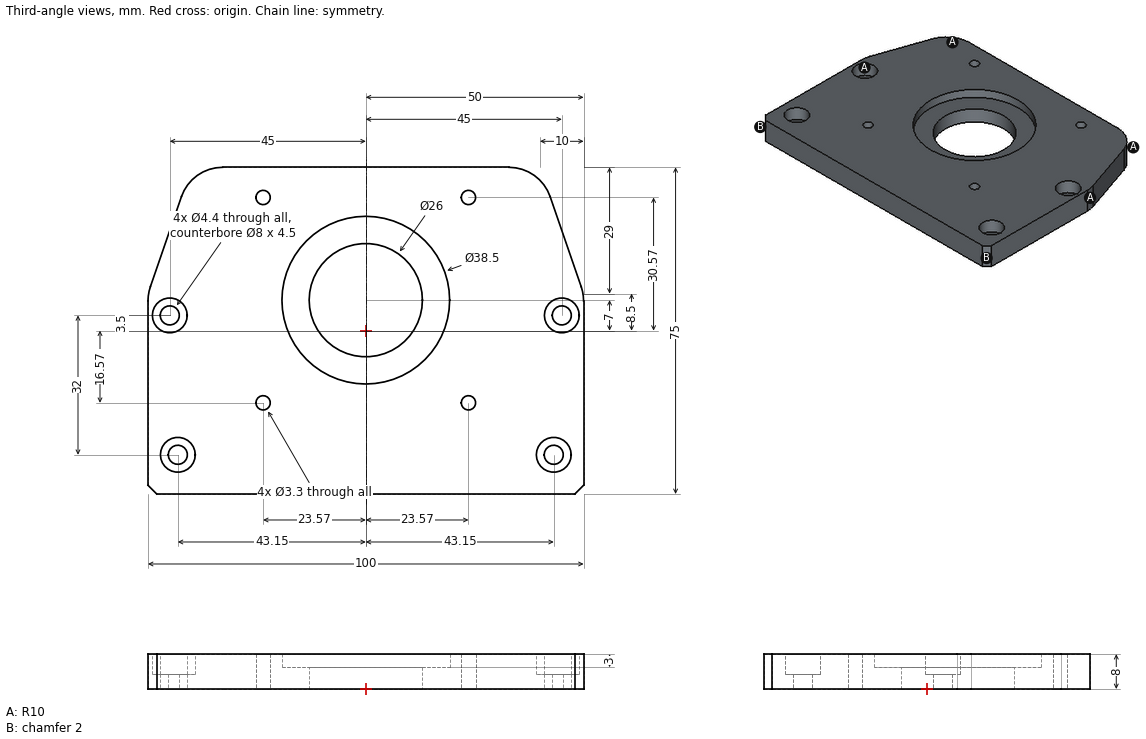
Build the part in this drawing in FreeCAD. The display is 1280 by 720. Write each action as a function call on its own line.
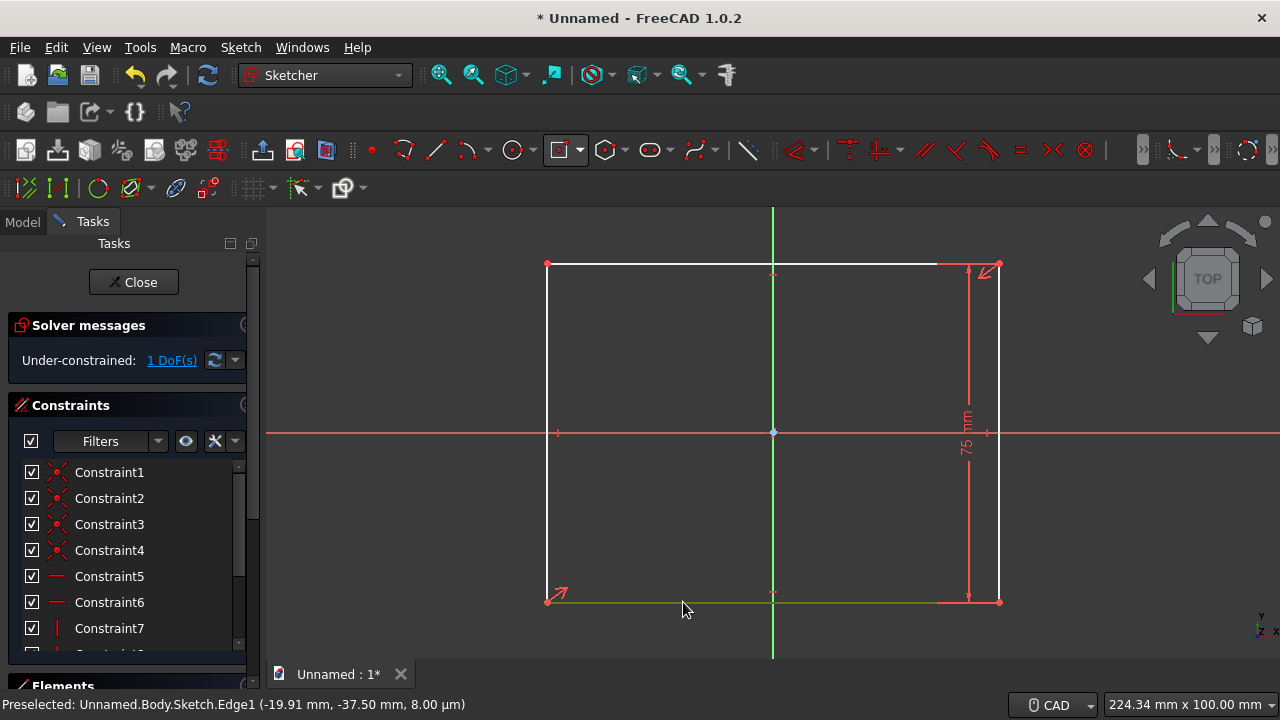
key(l)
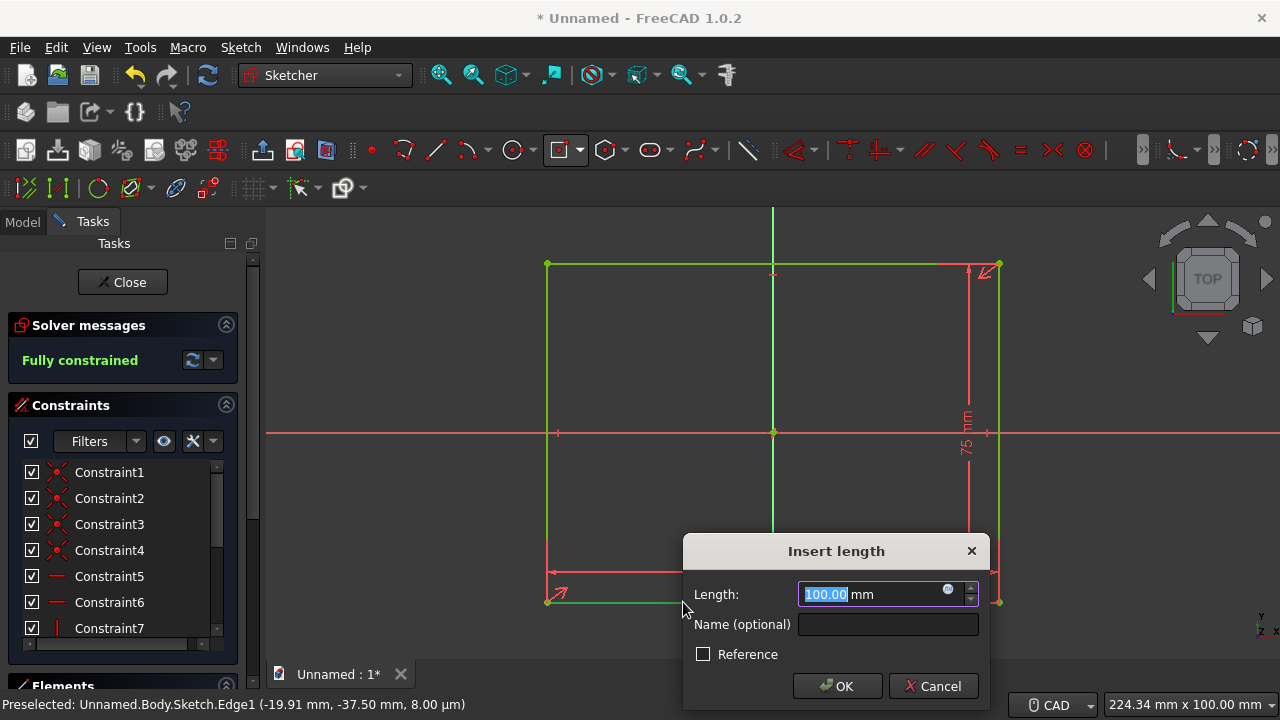
text(100)
key(Return)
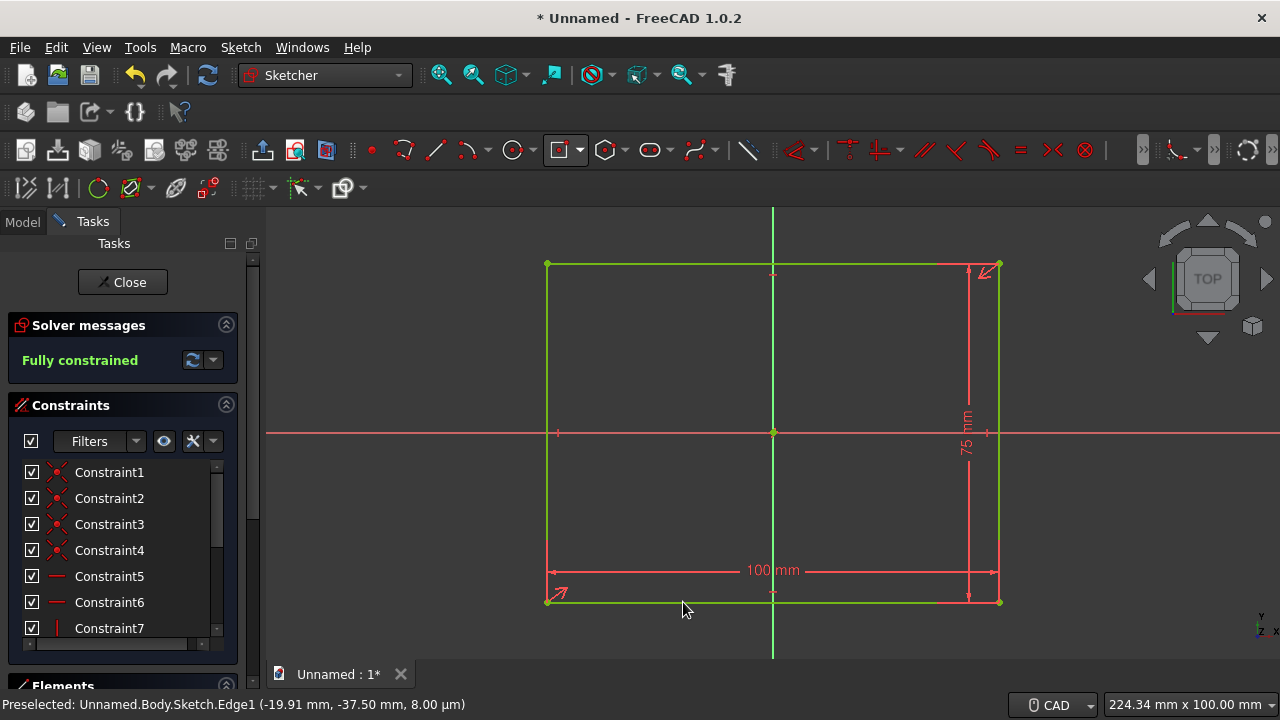
click(123, 282)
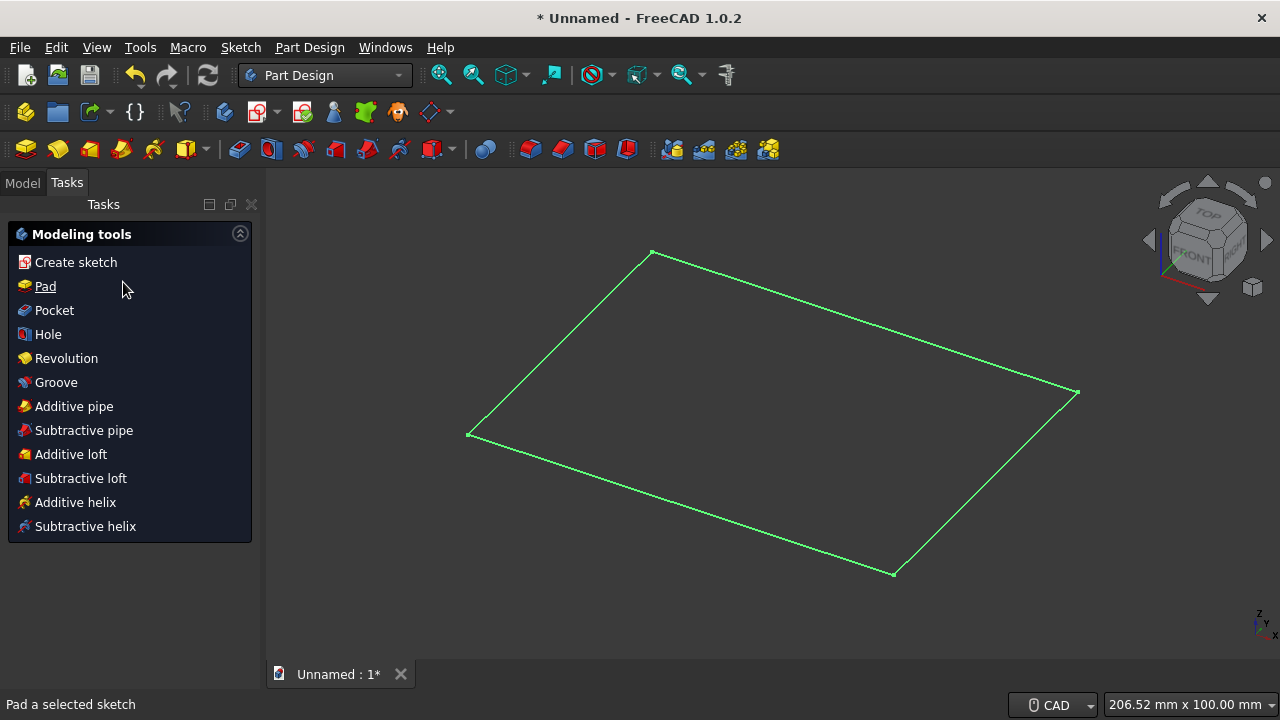
click(26, 150)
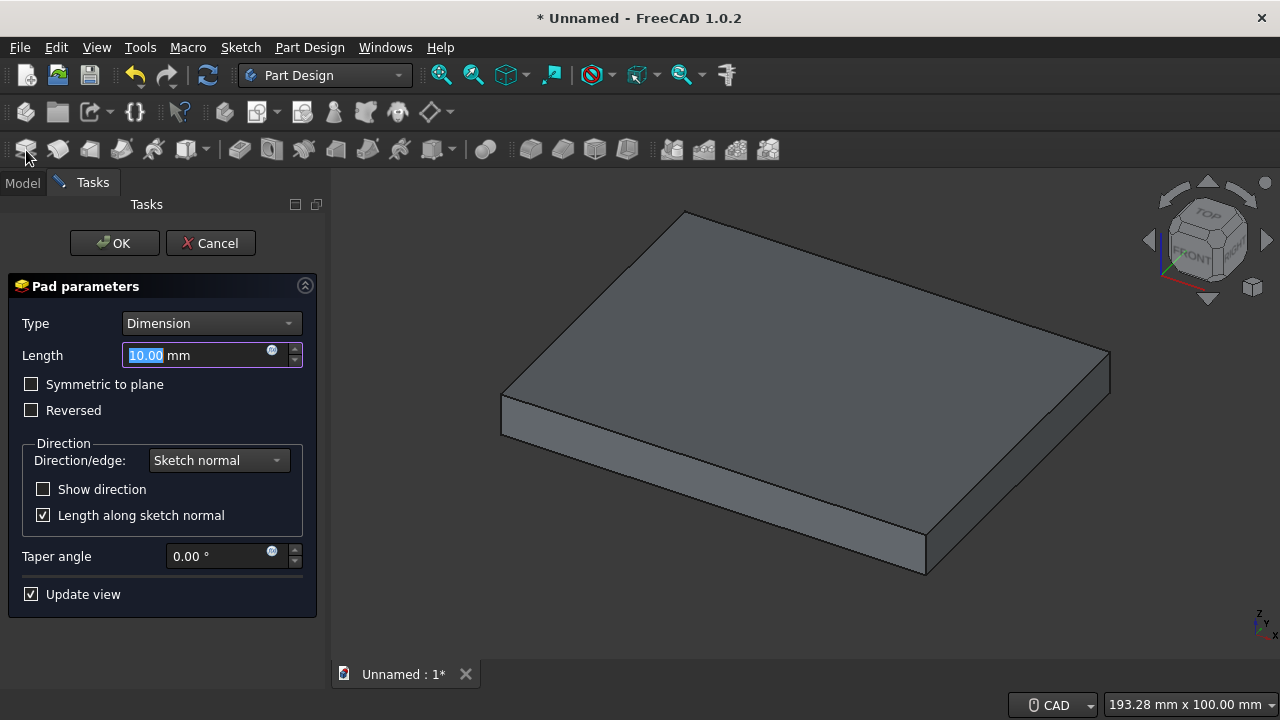
text(8)
key(Tab)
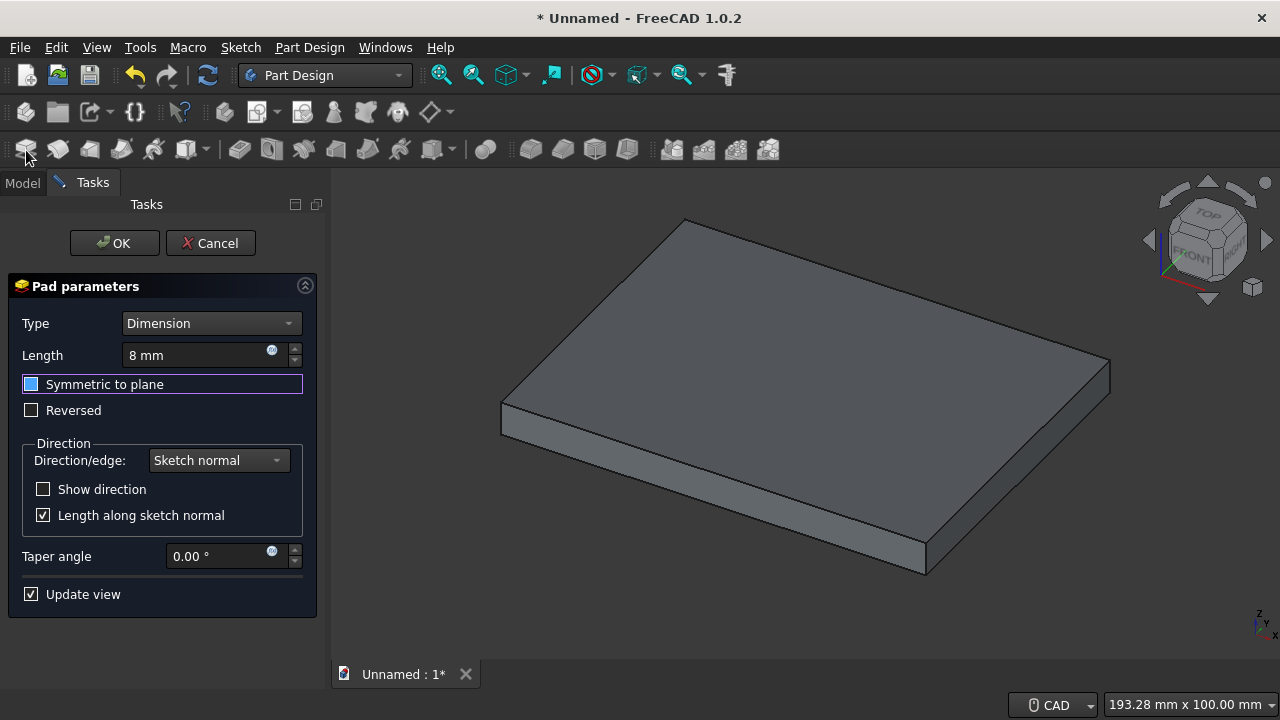
click(115, 243)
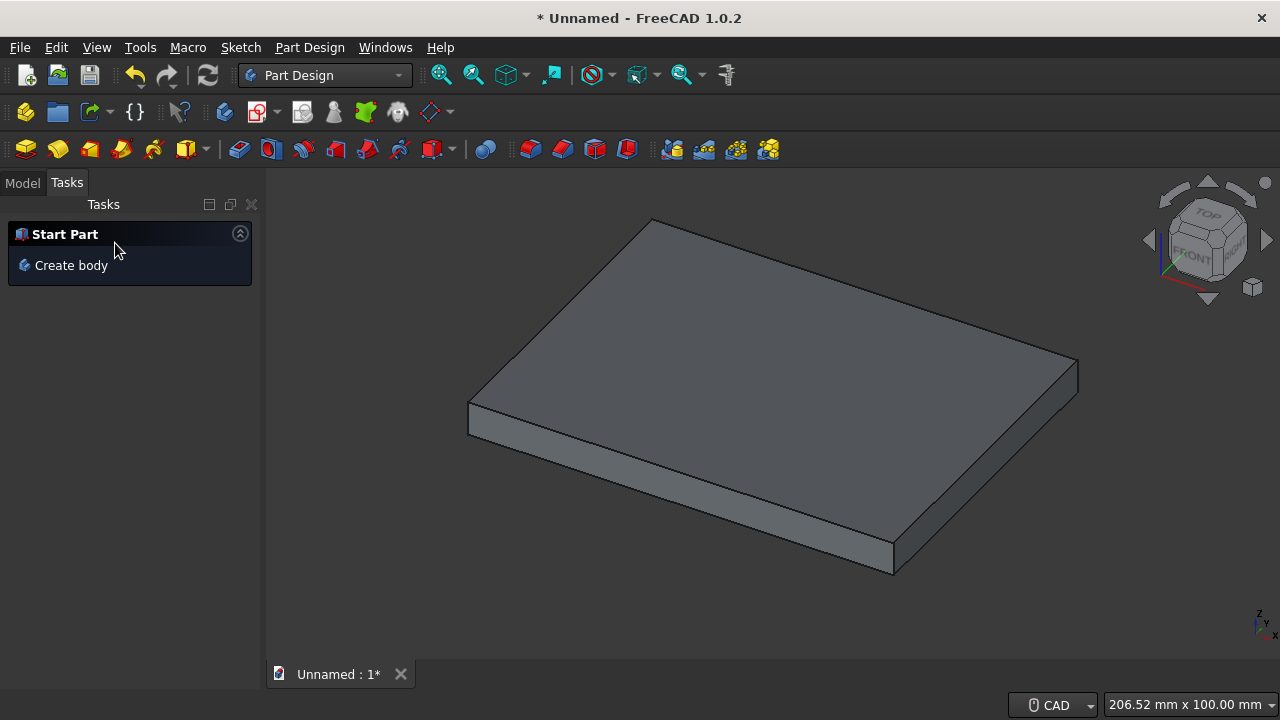
click(258, 112)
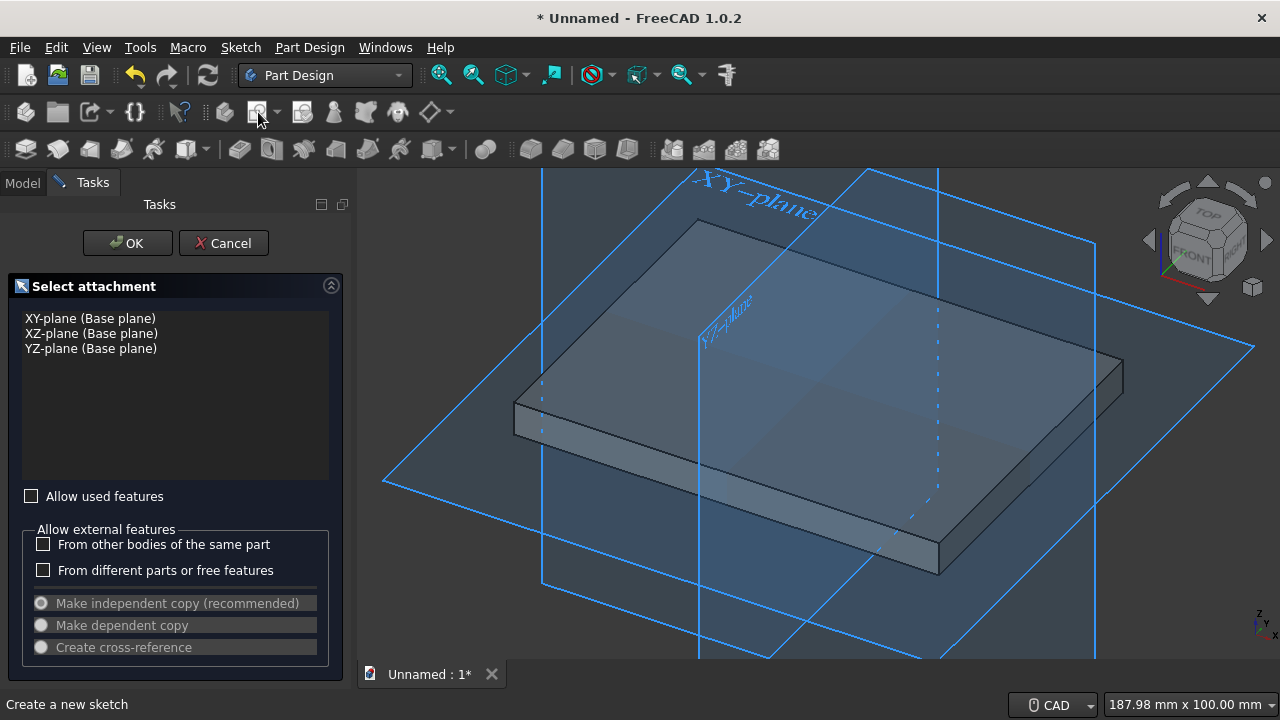
click(82, 318)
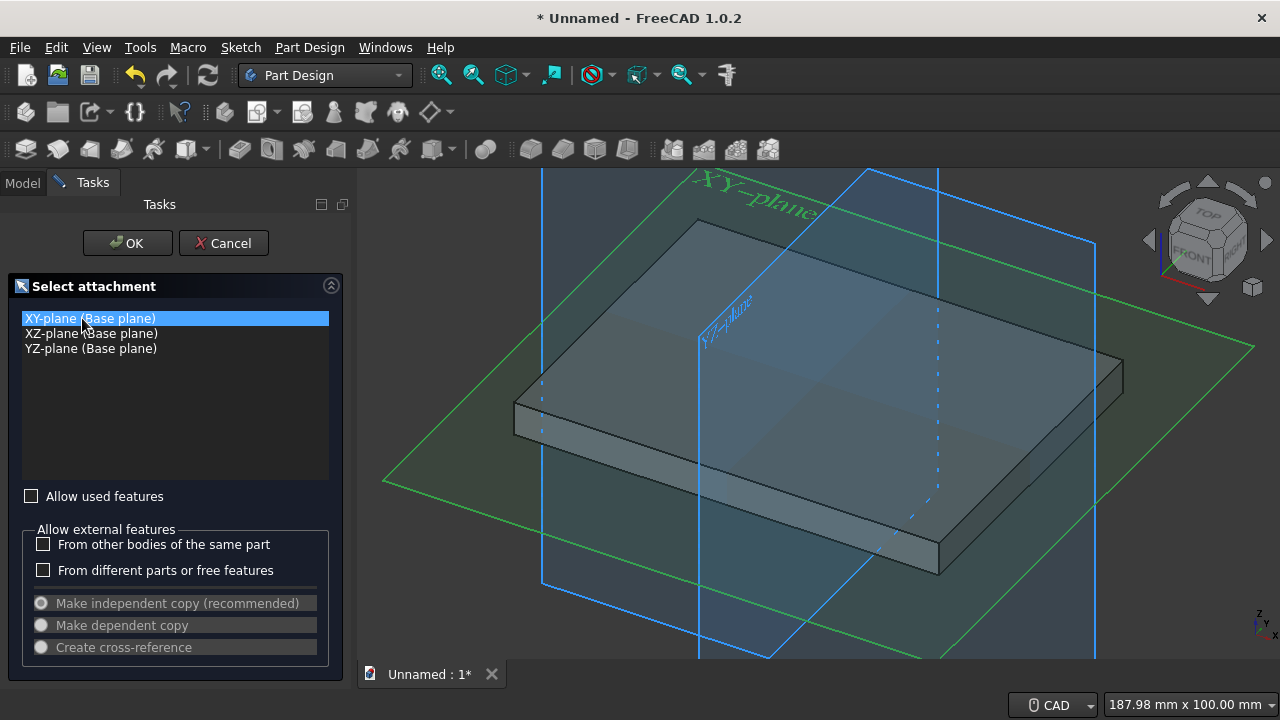
click(128, 243)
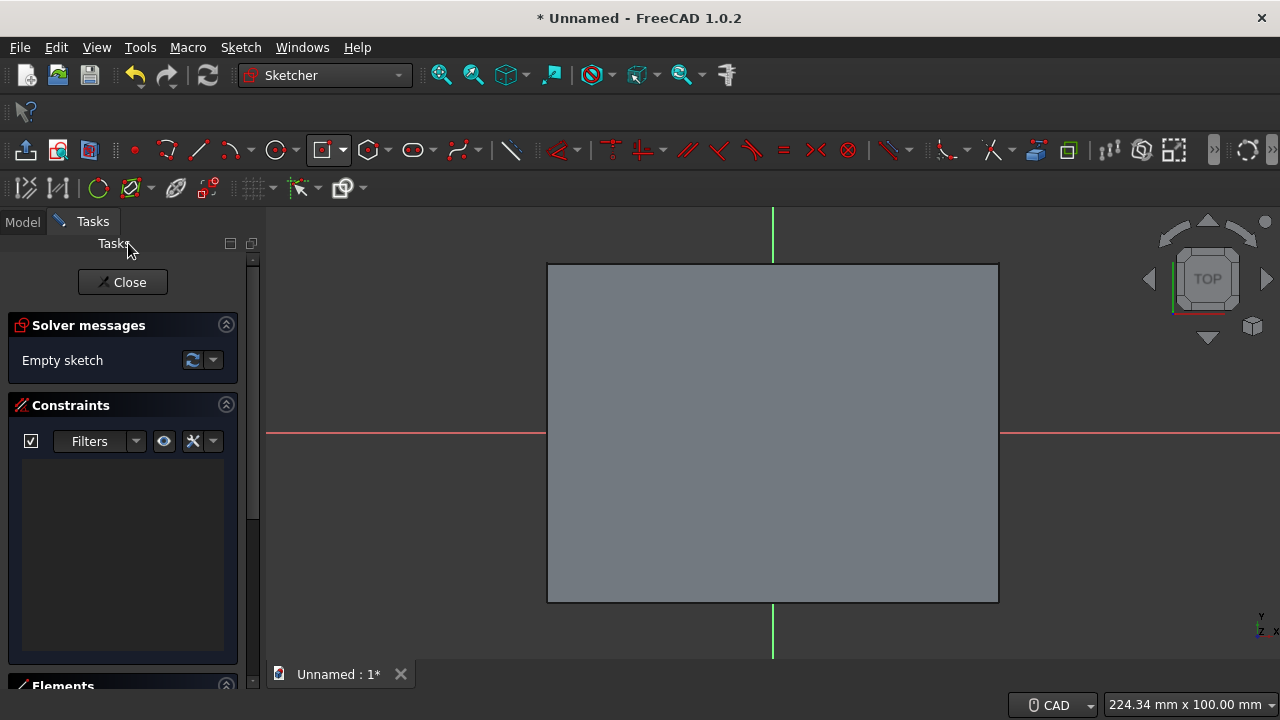
click(90, 150)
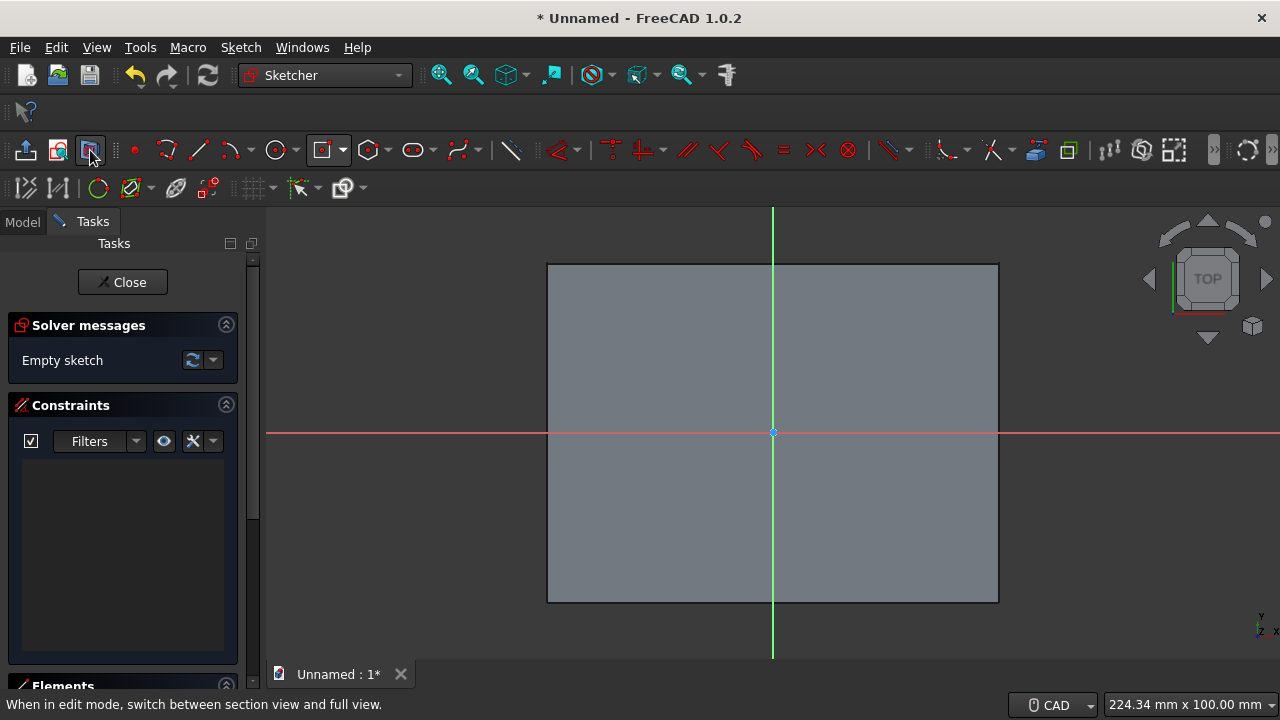
click(168, 150)